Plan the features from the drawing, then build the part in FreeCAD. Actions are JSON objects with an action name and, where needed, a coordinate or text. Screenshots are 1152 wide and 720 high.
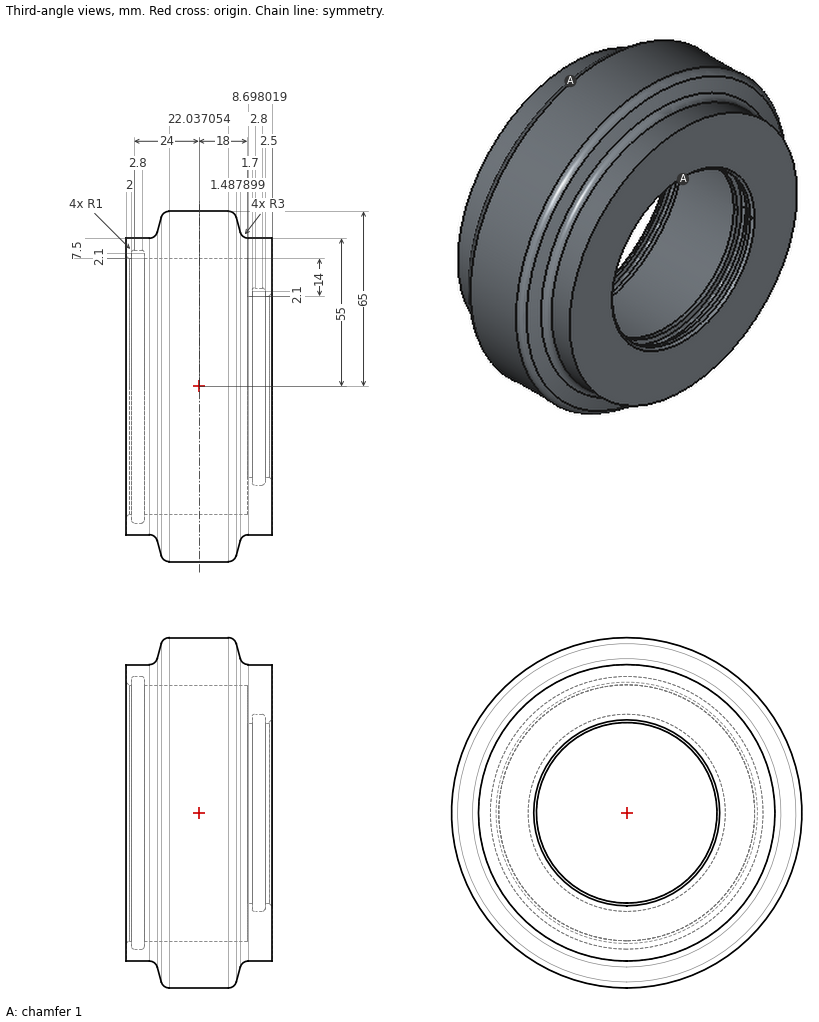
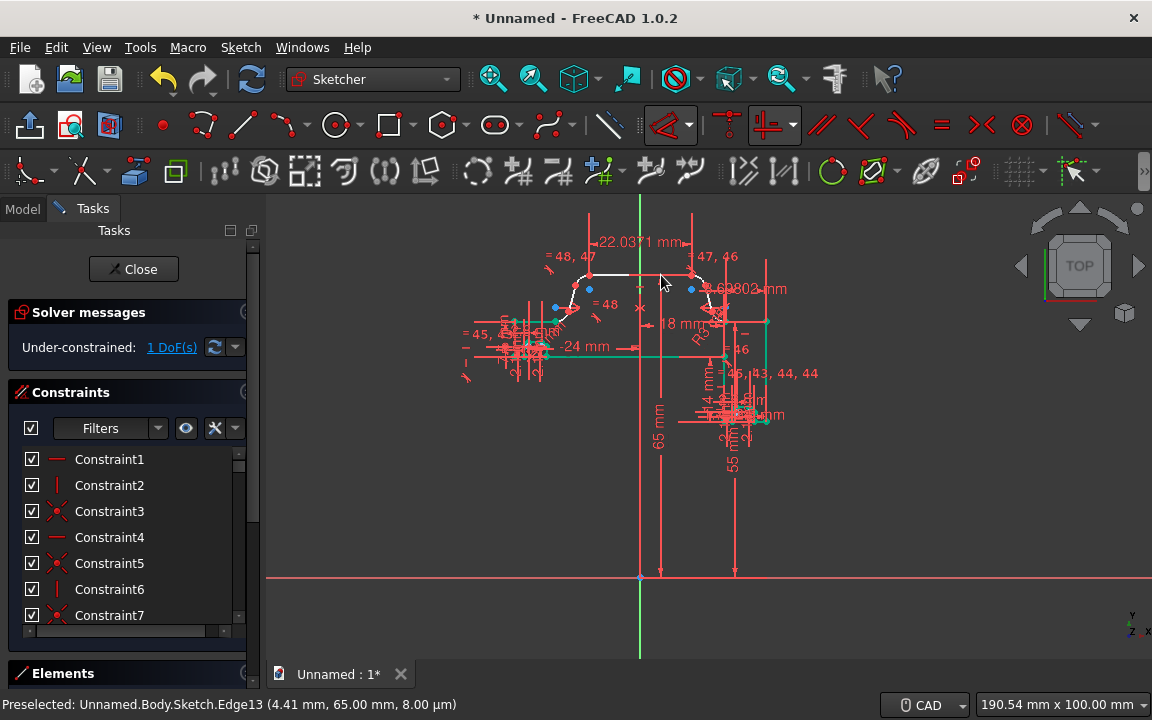
{"action": "scroll", "coordinate": [709, 301], "scroll_direction": "up", "scroll_amount": 9}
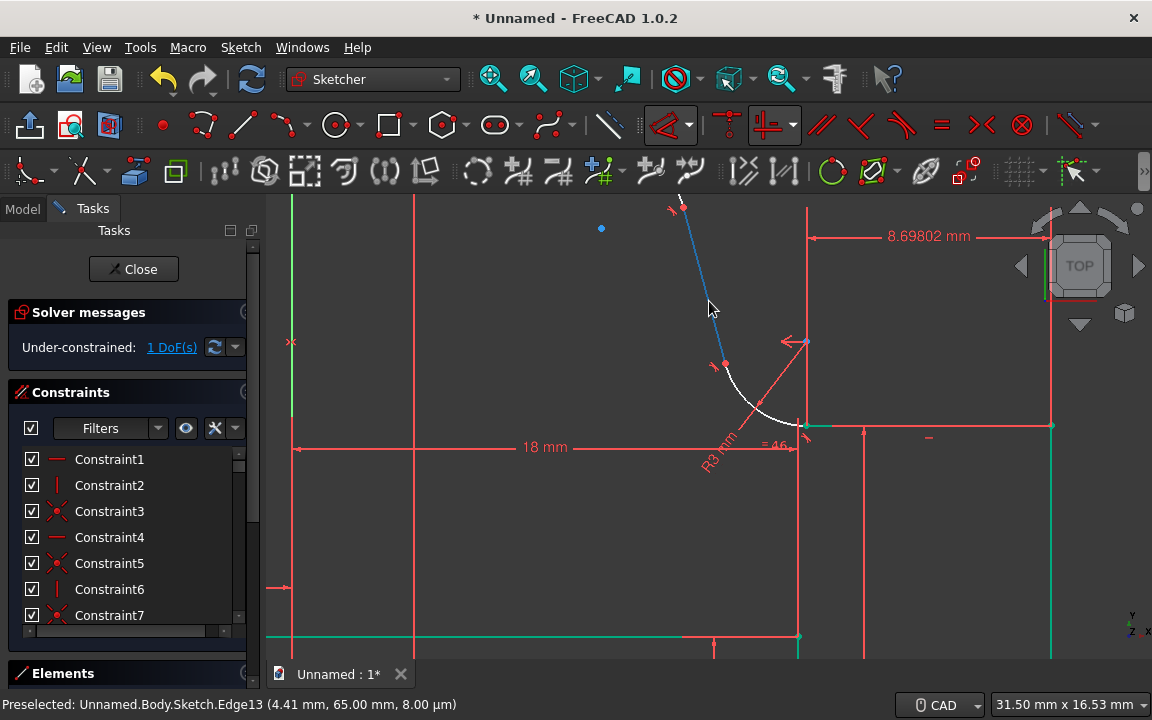
{"action": "left_click", "coordinate": [708, 301]}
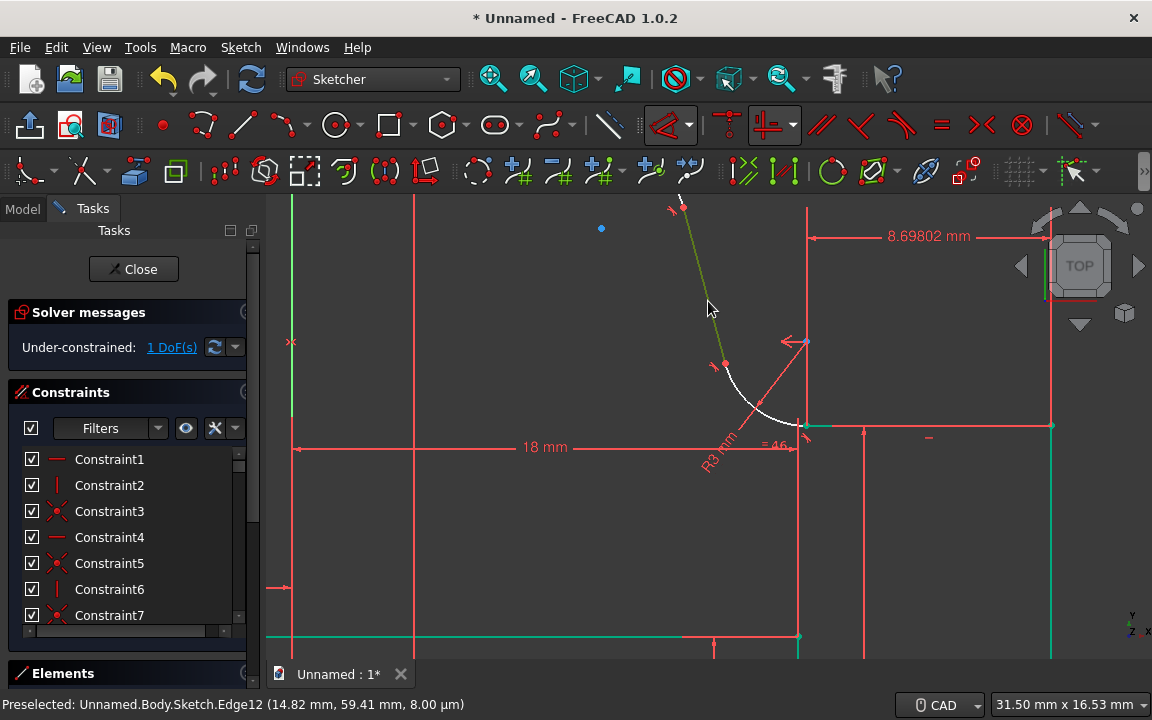
{"action": "key", "text": "l"}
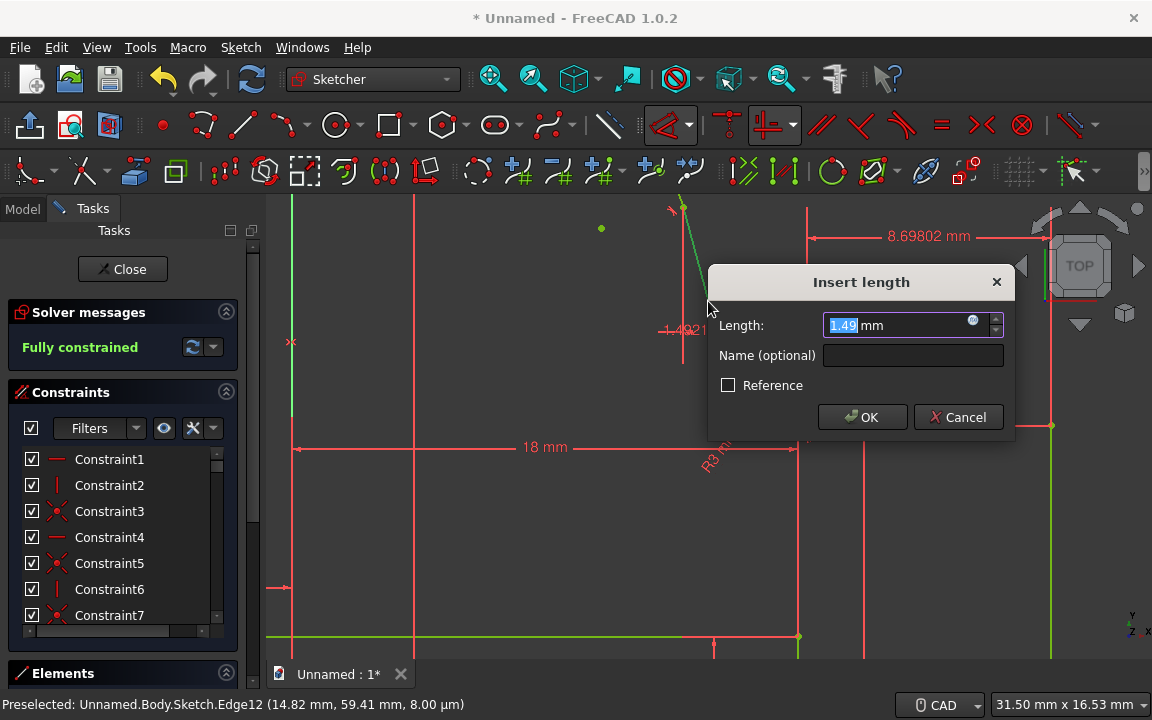
{"action": "type", "text": "1.487899"}
{"action": "key", "text": "Return"}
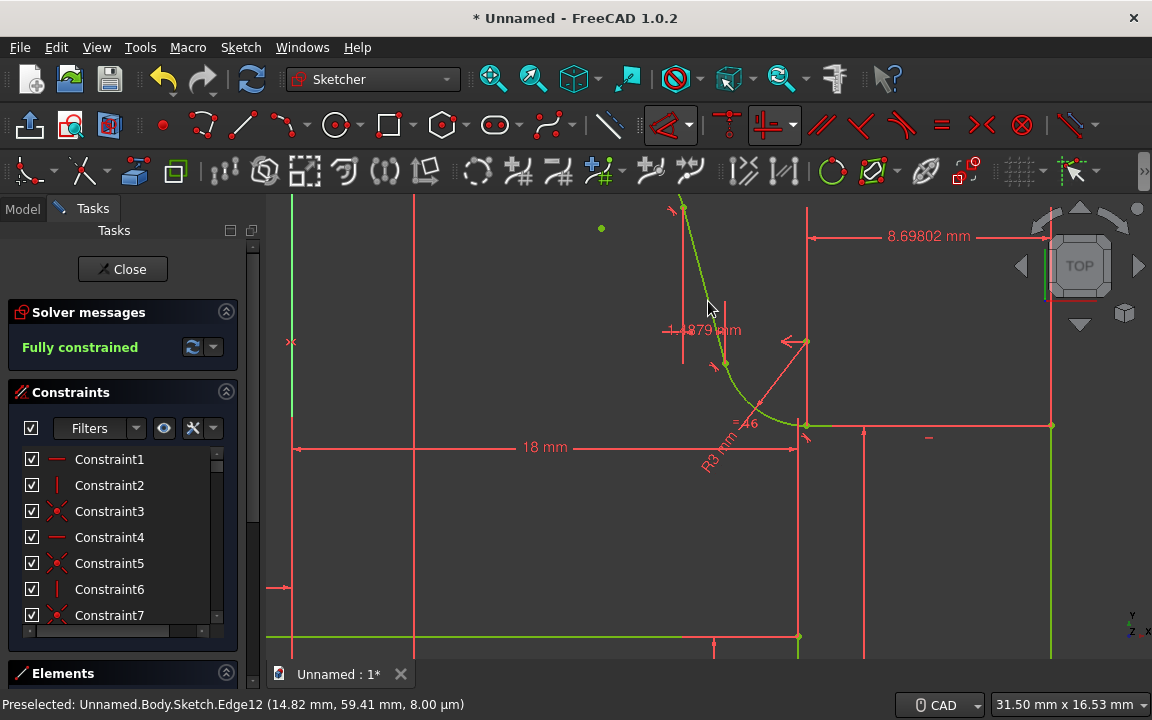
{"action": "left_click", "coordinate": [123, 269]}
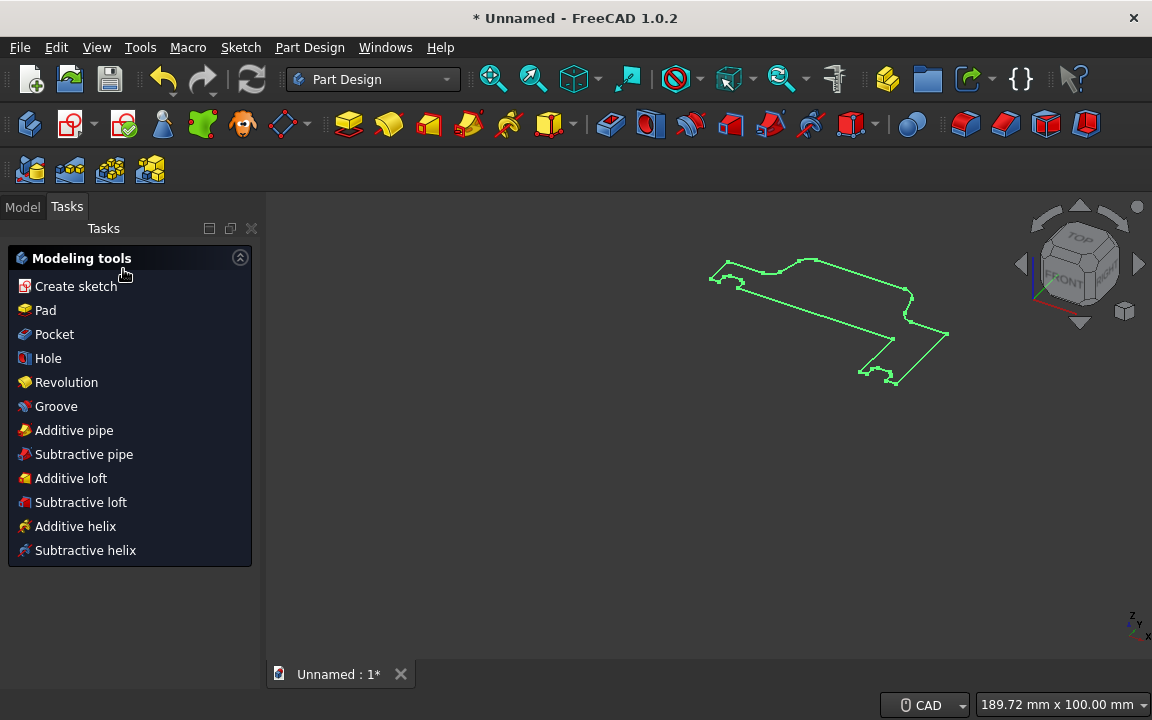
{"action": "left_click", "coordinate": [390, 124]}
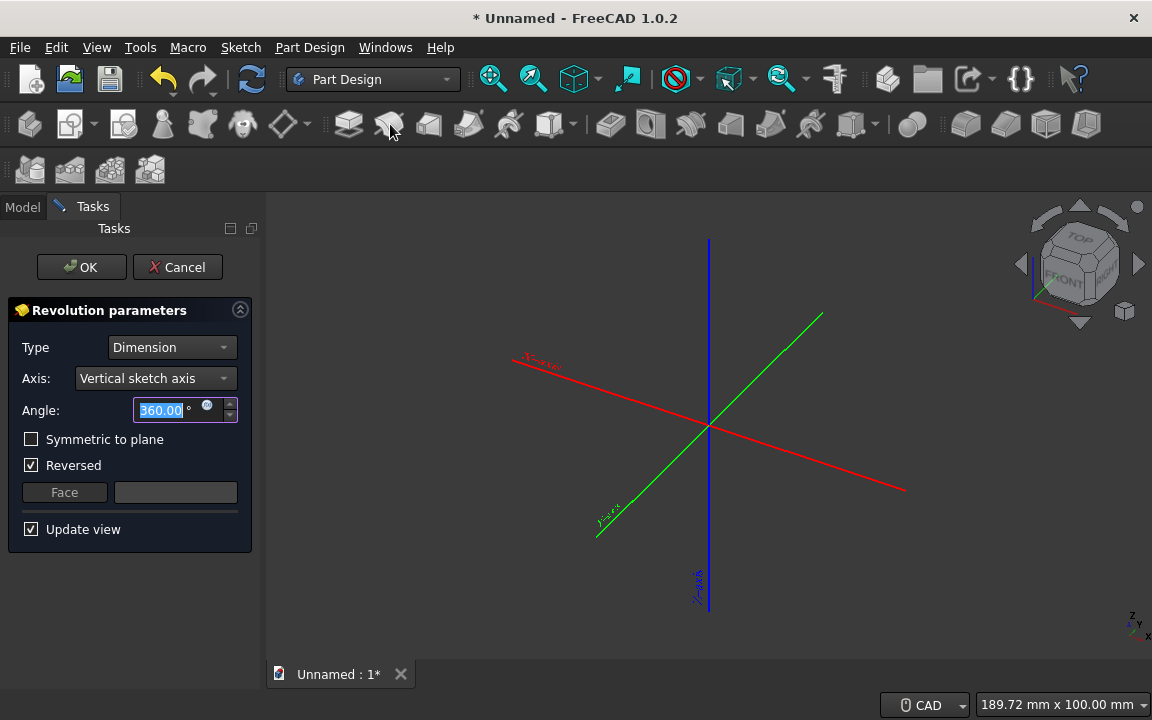
{"action": "left_click", "coordinate": [156, 378]}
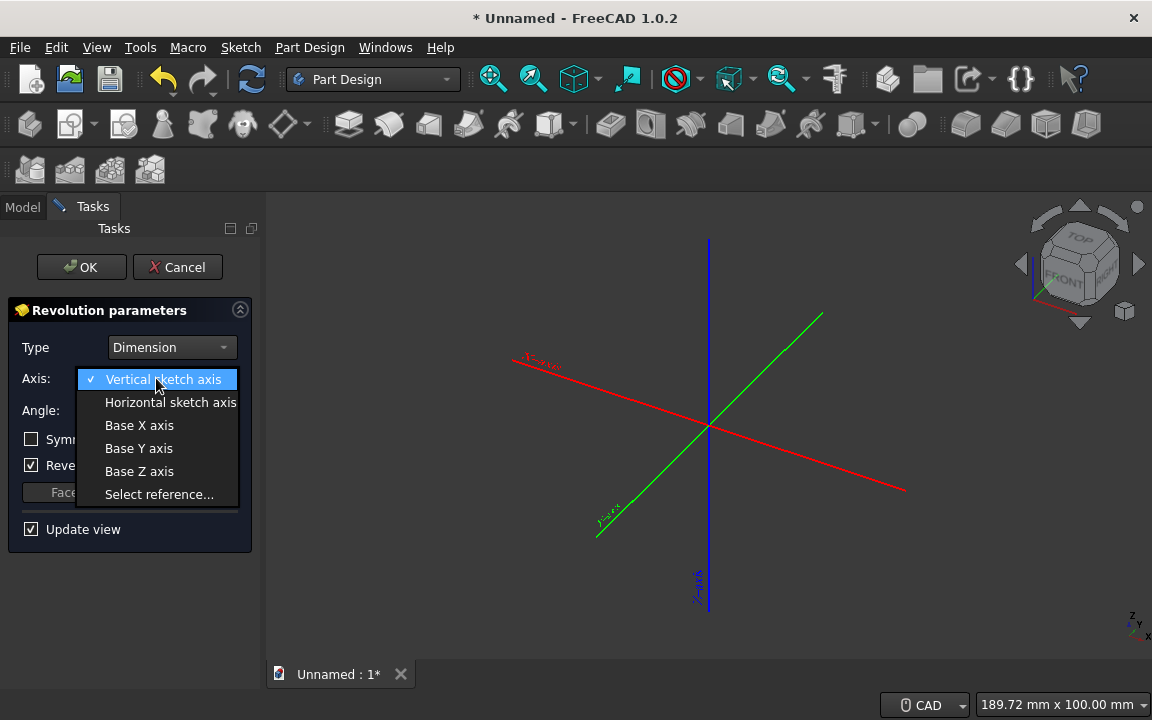
{"action": "left_click", "coordinate": [156, 402]}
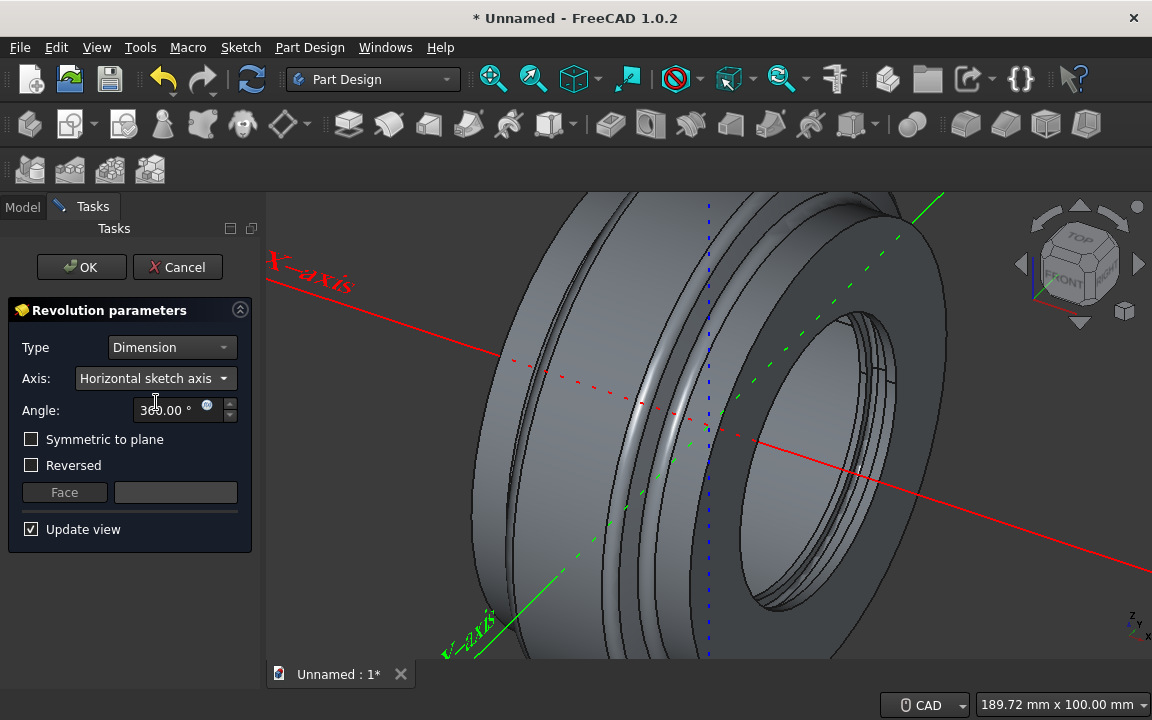
{"action": "left_click", "coordinate": [82, 267]}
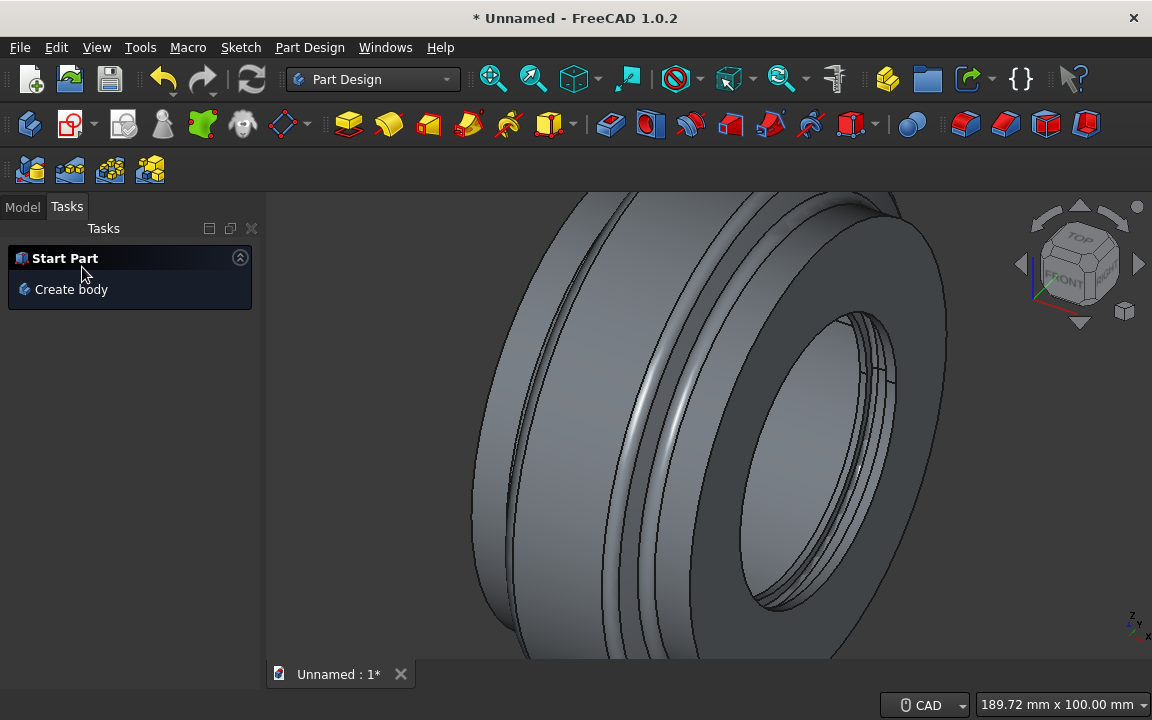
{"action": "key", "text": "v f"}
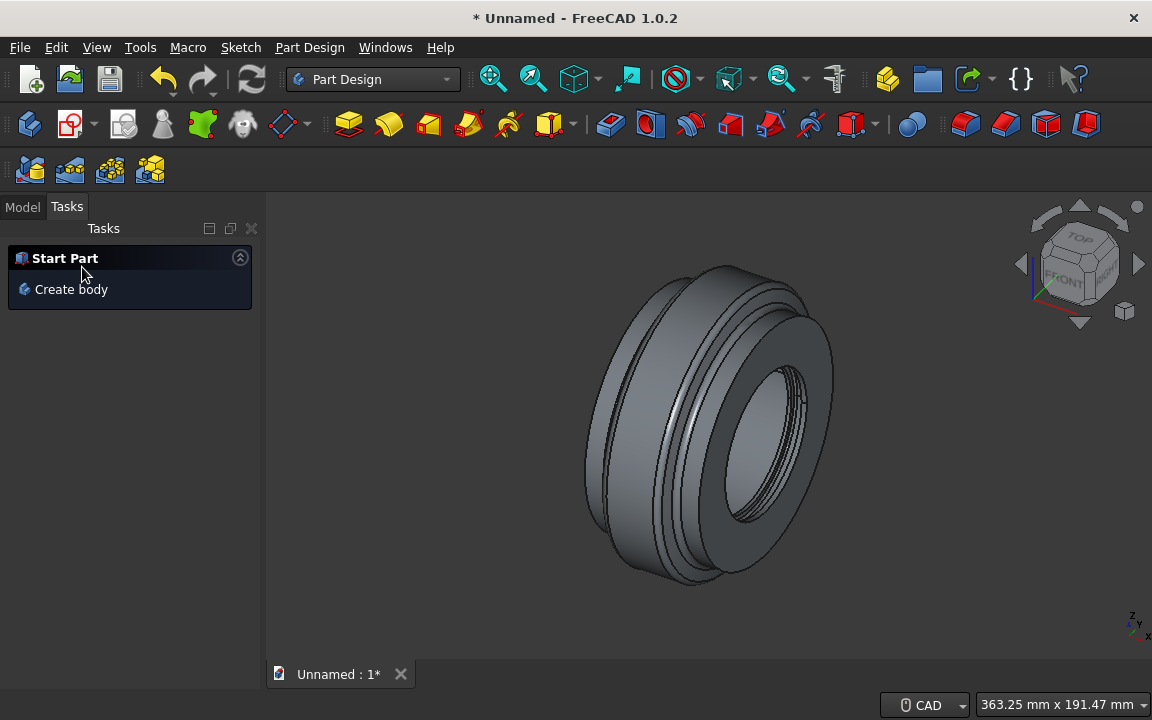
{"action": "left_click", "coordinate": [753, 520]}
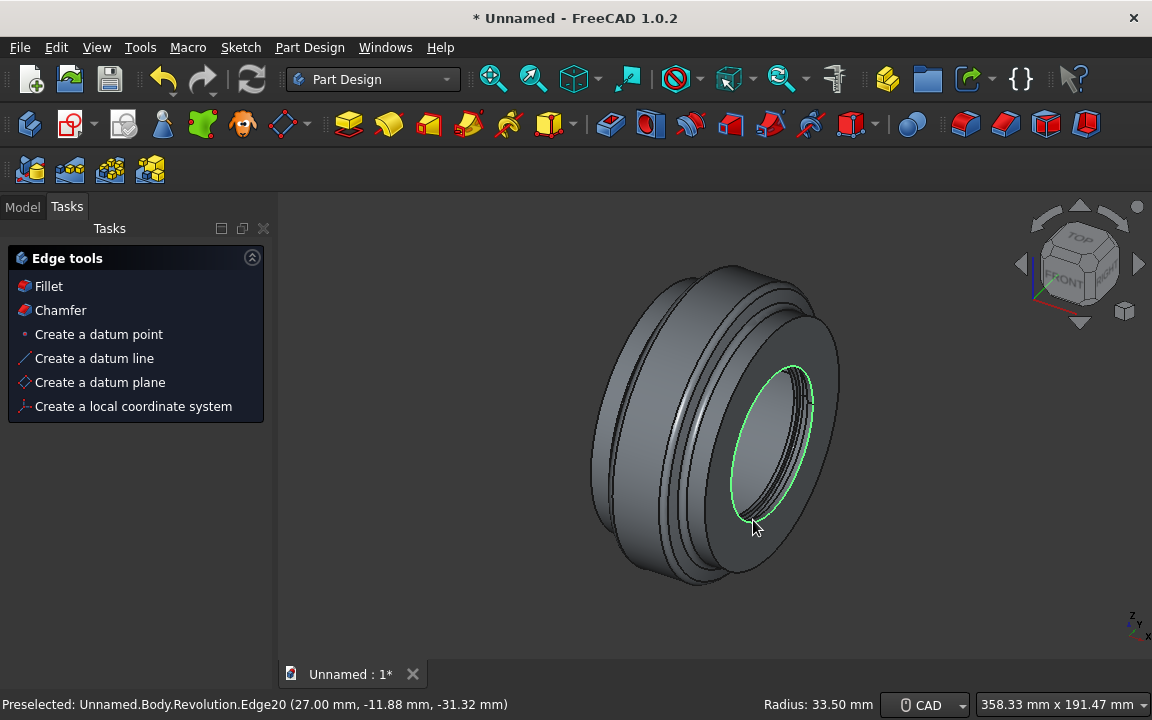
{"action": "key", "text": "0"}